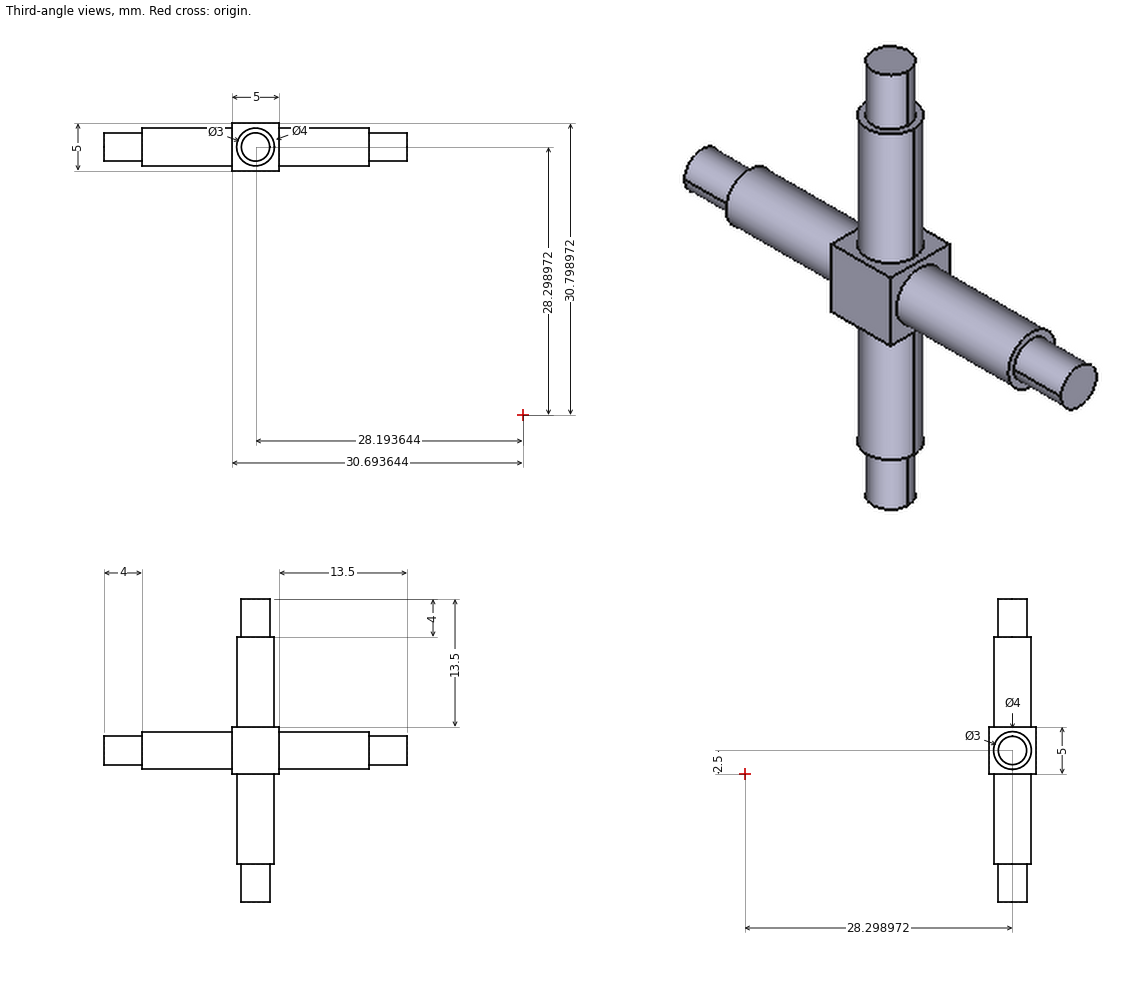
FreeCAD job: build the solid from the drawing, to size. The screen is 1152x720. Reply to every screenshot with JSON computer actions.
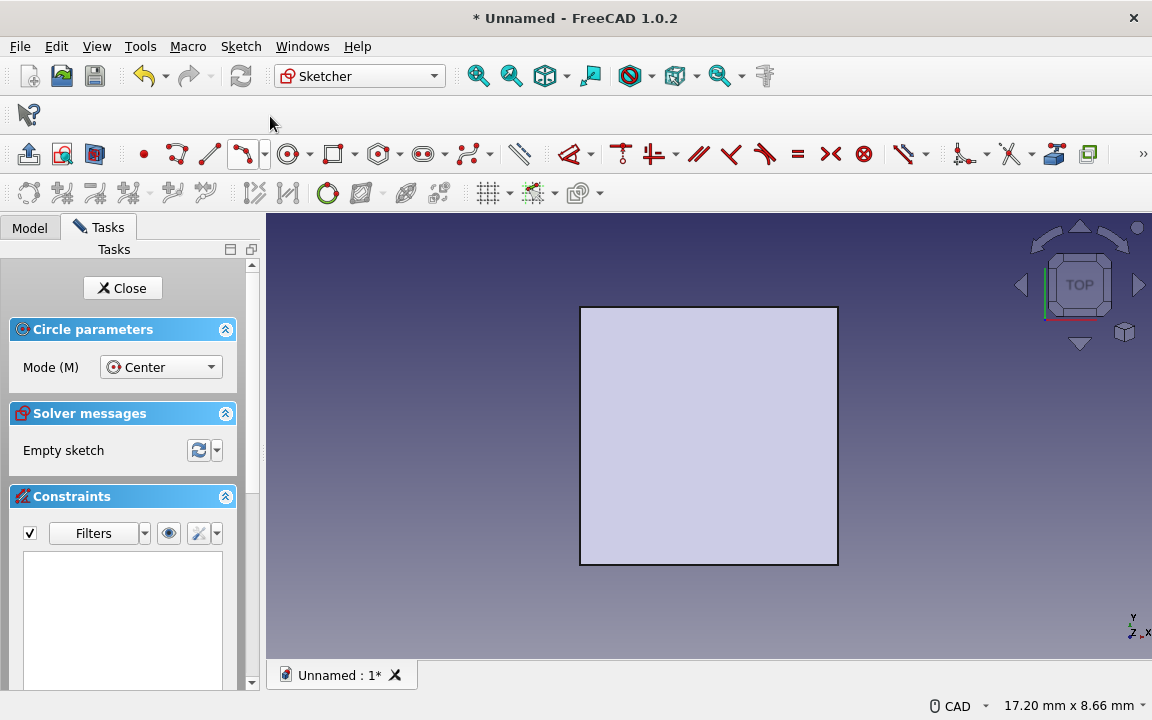
{"action": "left_click", "coordinate": [709, 436]}
{"action": "left_click", "coordinate": [782, 363]}
{"action": "key", "text": "Escape"}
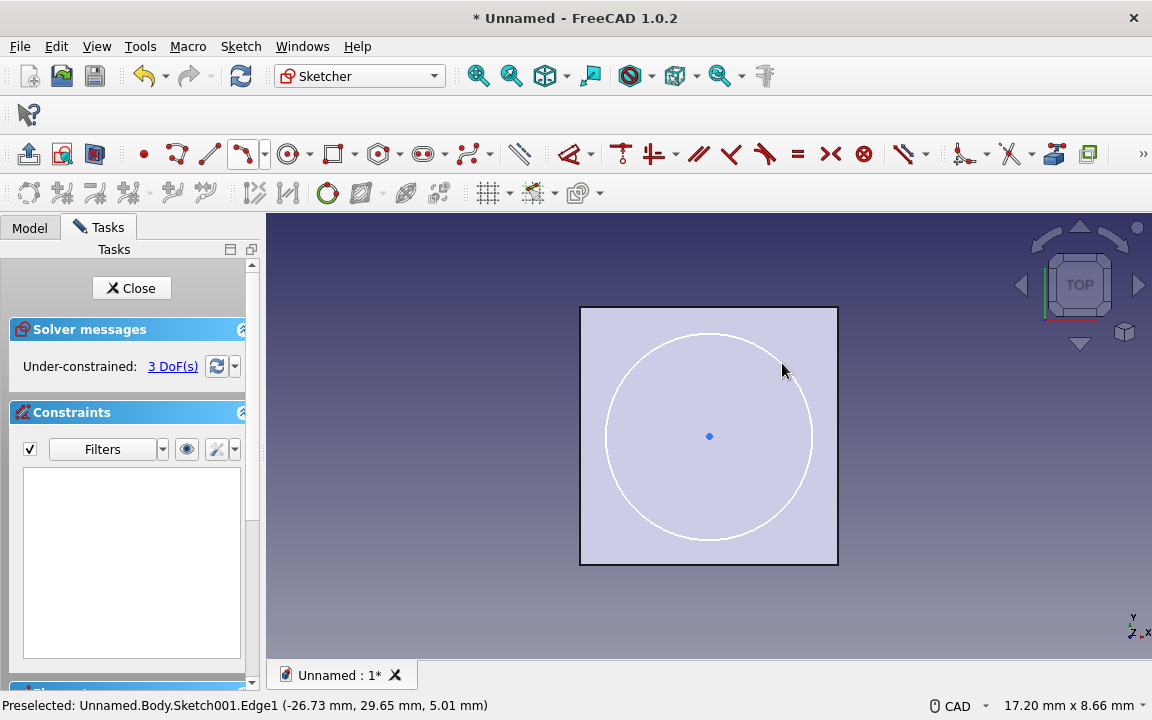
{"action": "left_click", "coordinate": [568, 154]}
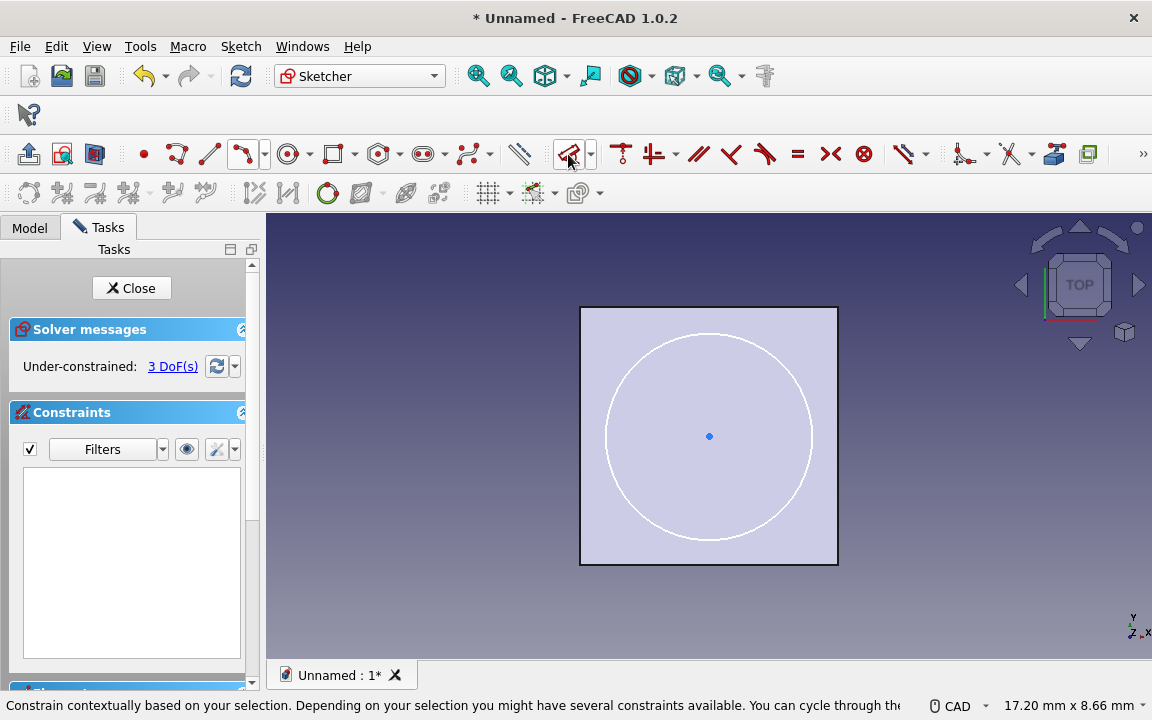
{"action": "left_click", "coordinate": [782, 364]}
{"action": "left_click", "coordinate": [805, 341]}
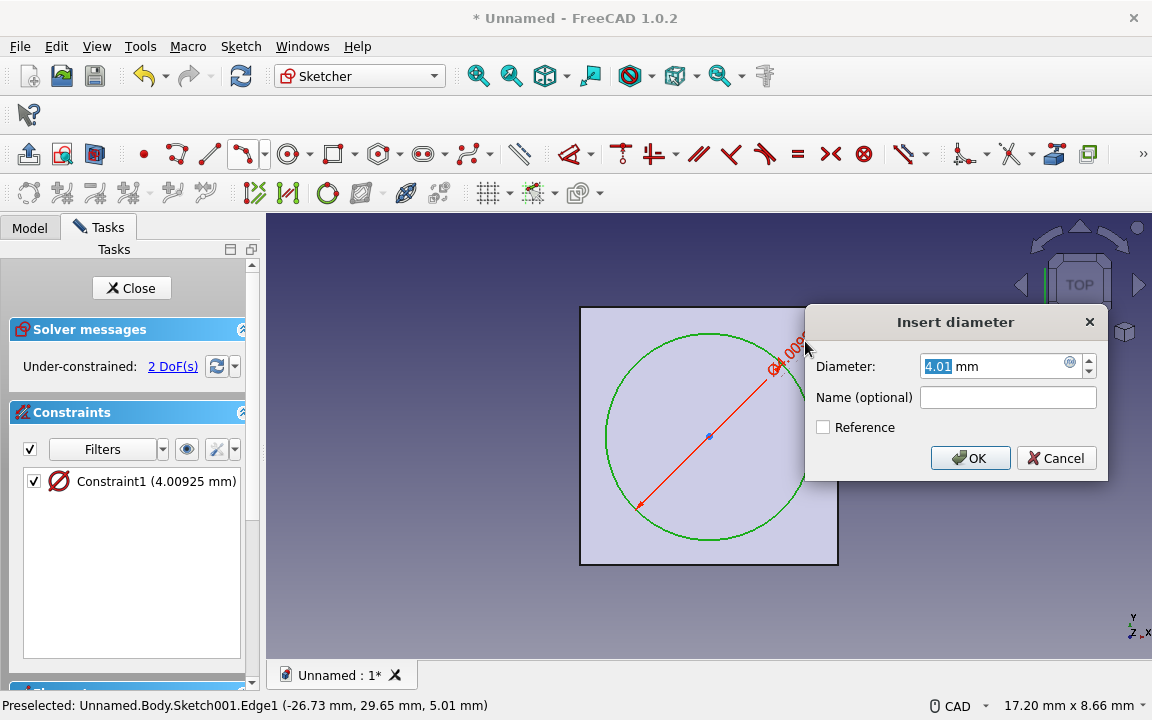
{"action": "type", "text": "4"}
{"action": "key", "text": "Return"}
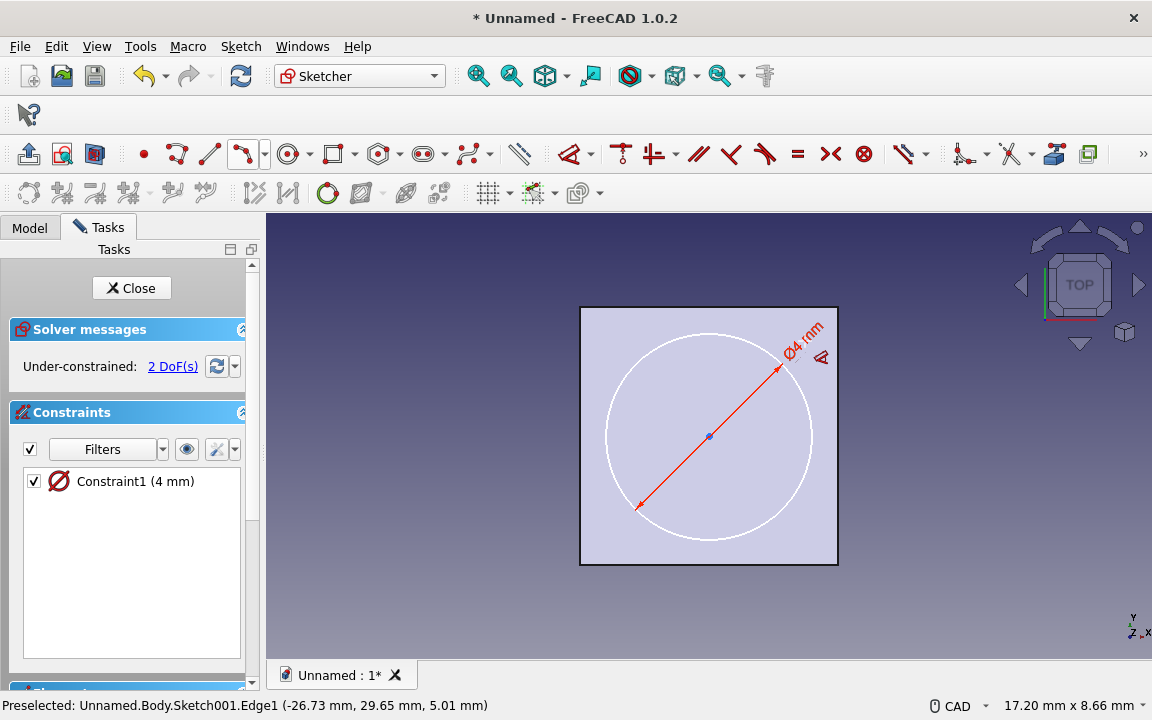
{"action": "left_click", "coordinate": [709, 437]}
{"action": "left_click", "coordinate": [848, 403]}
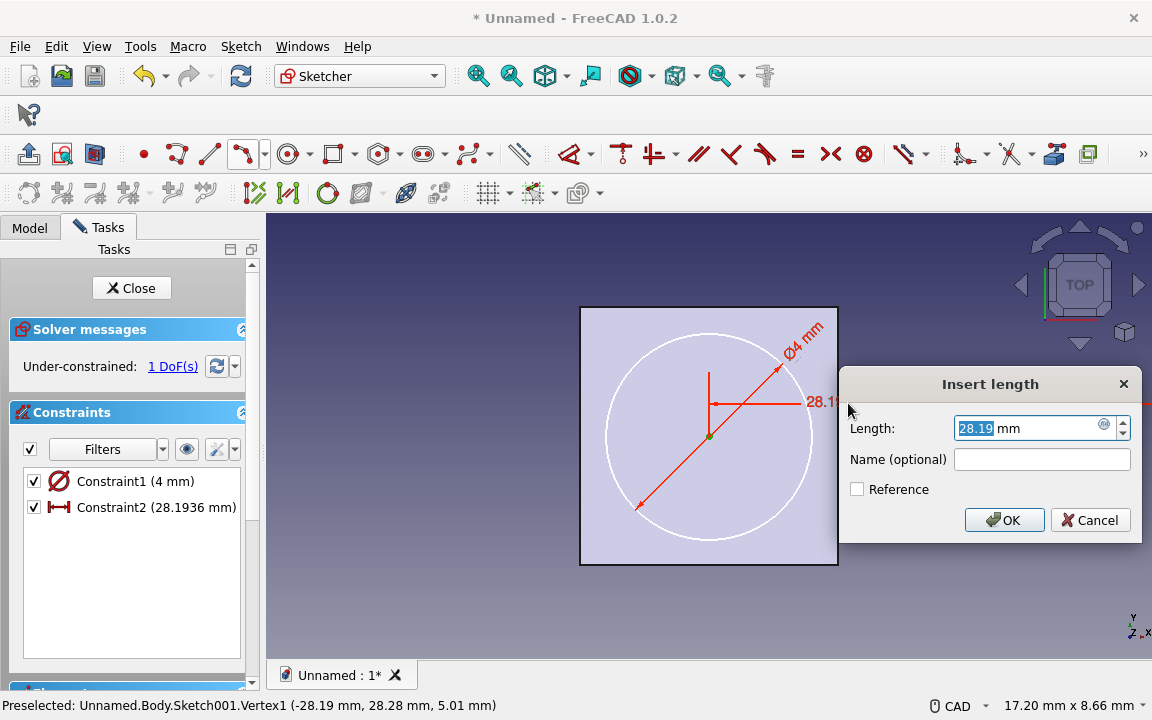
{"action": "type", "text": "28.193644"}
{"action": "key", "text": "Return"}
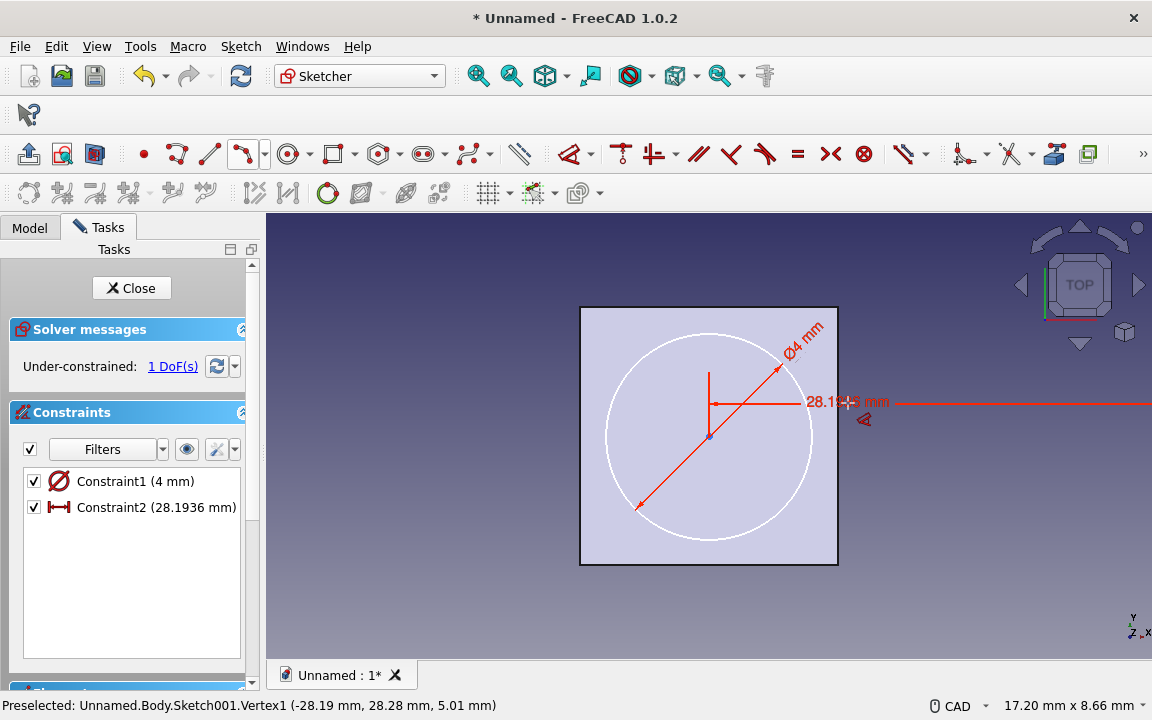
{"action": "left_click", "coordinate": [709, 437]}
{"action": "left_click", "coordinate": [675, 489]}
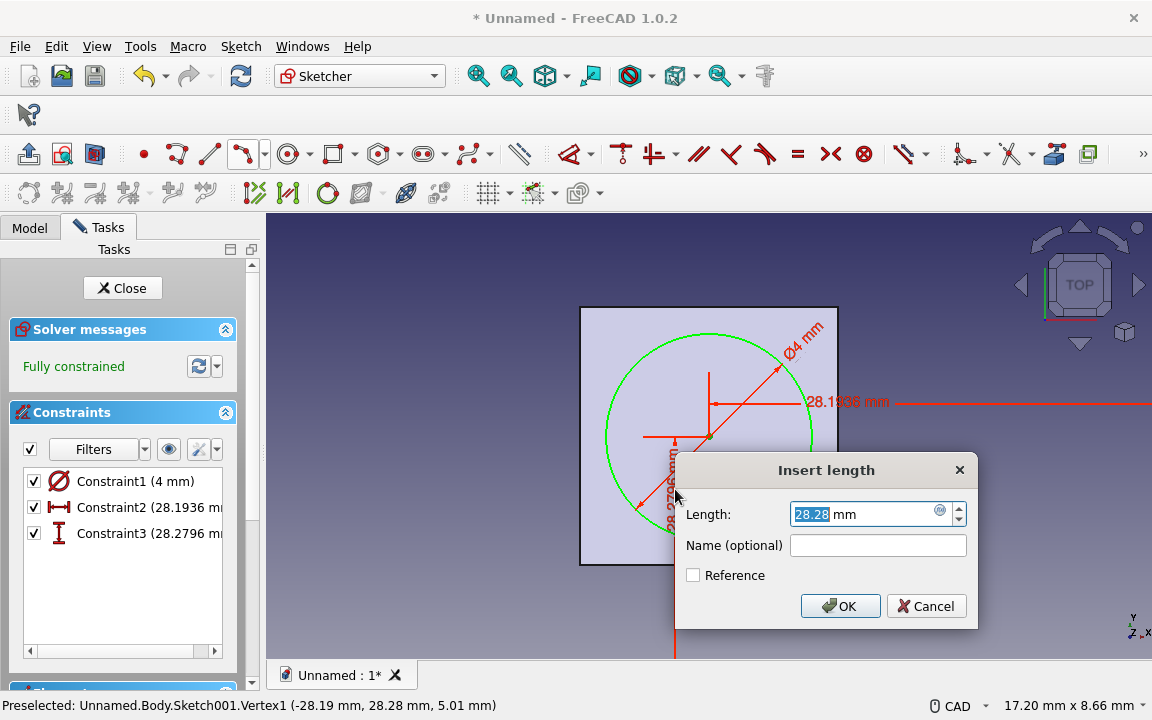
{"action": "type", "text": "28.298972"}
{"action": "key", "text": "Return"}
{"action": "key", "text": "Escape"}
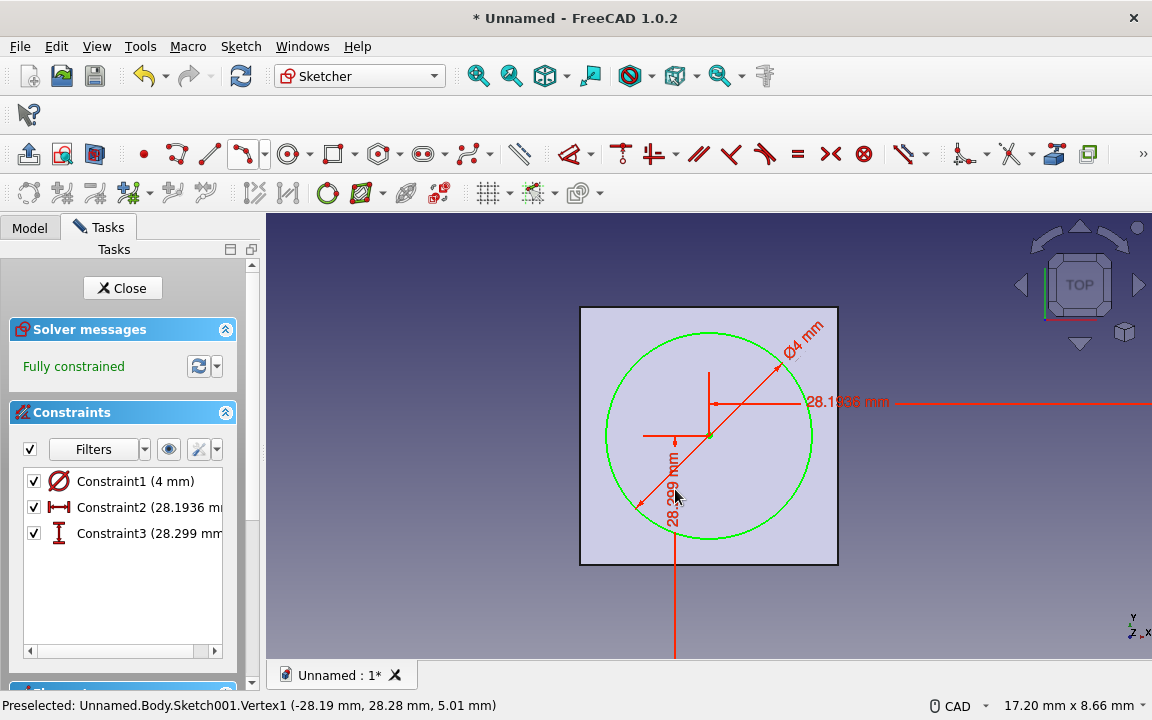
{"action": "left_click", "coordinate": [123, 288]}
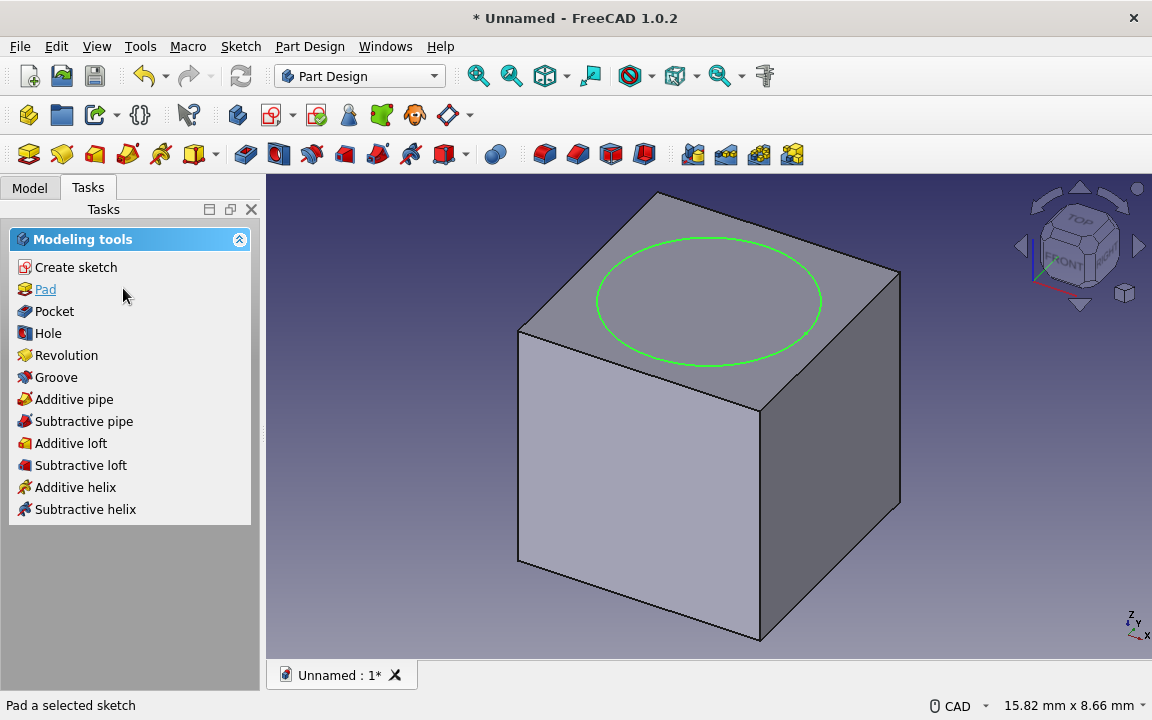
{"action": "left_click", "coordinate": [29, 154]}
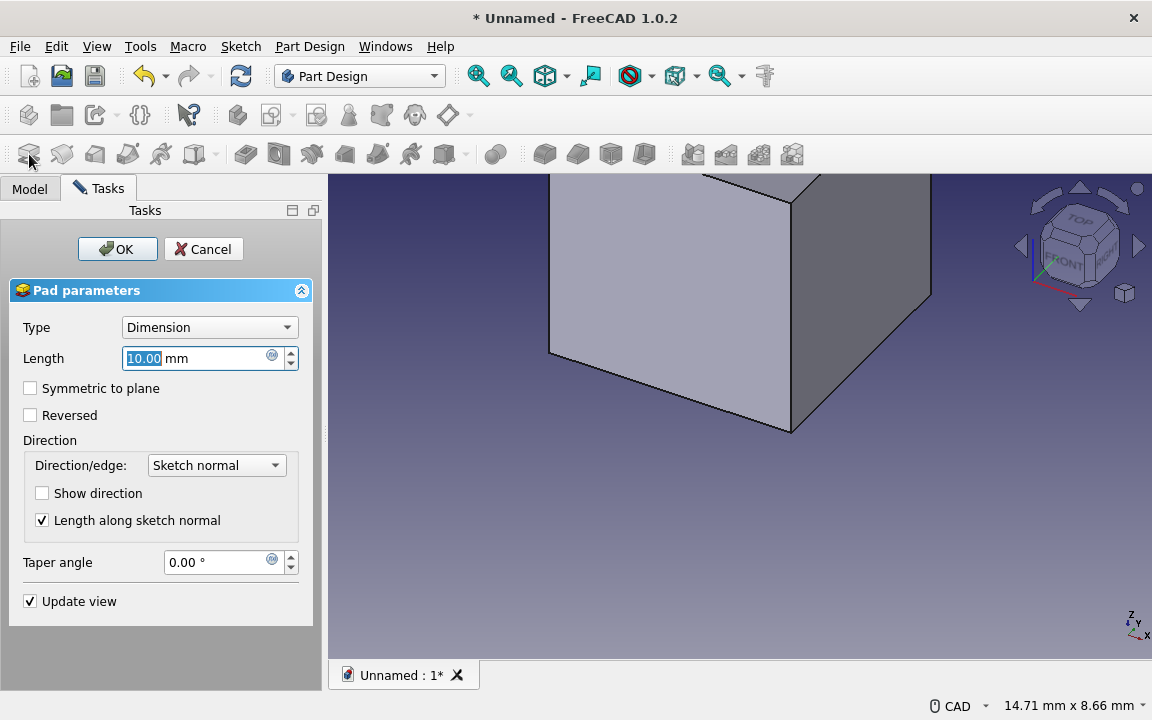
{"action": "type", "text": "13.5"}
{"action": "key", "text": "Tab"}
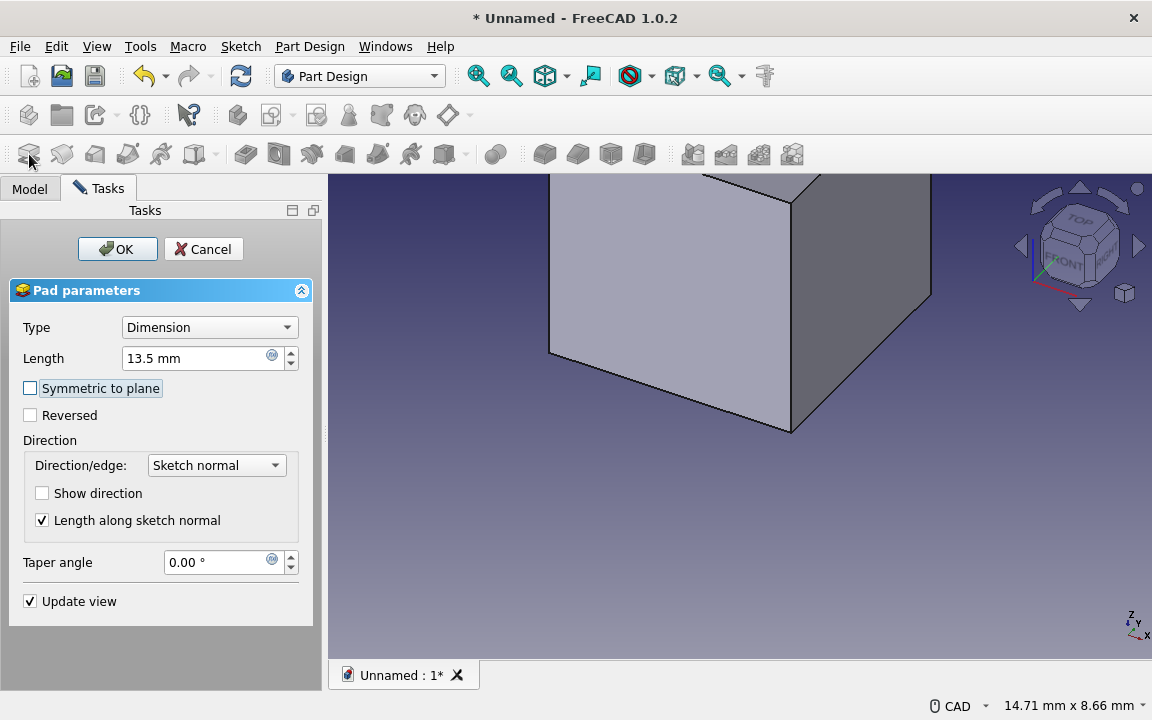
{"action": "left_click", "coordinate": [118, 249]}